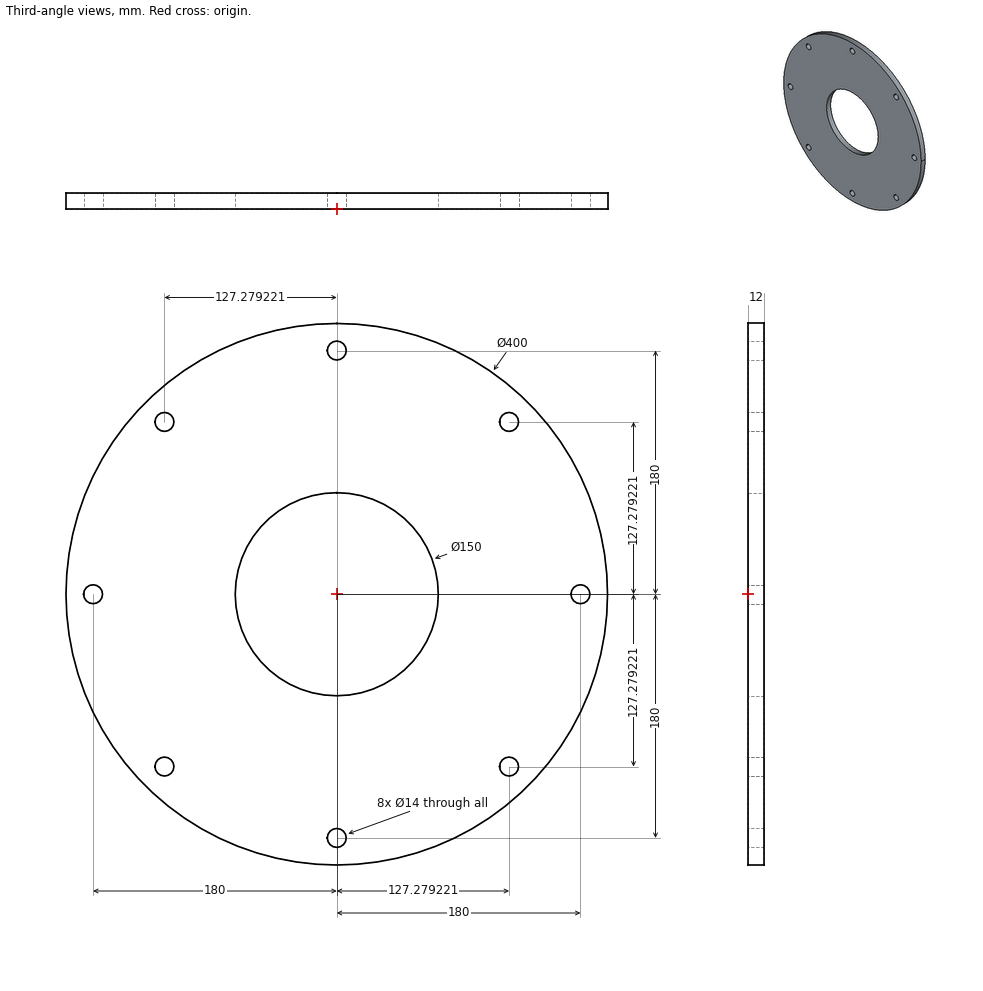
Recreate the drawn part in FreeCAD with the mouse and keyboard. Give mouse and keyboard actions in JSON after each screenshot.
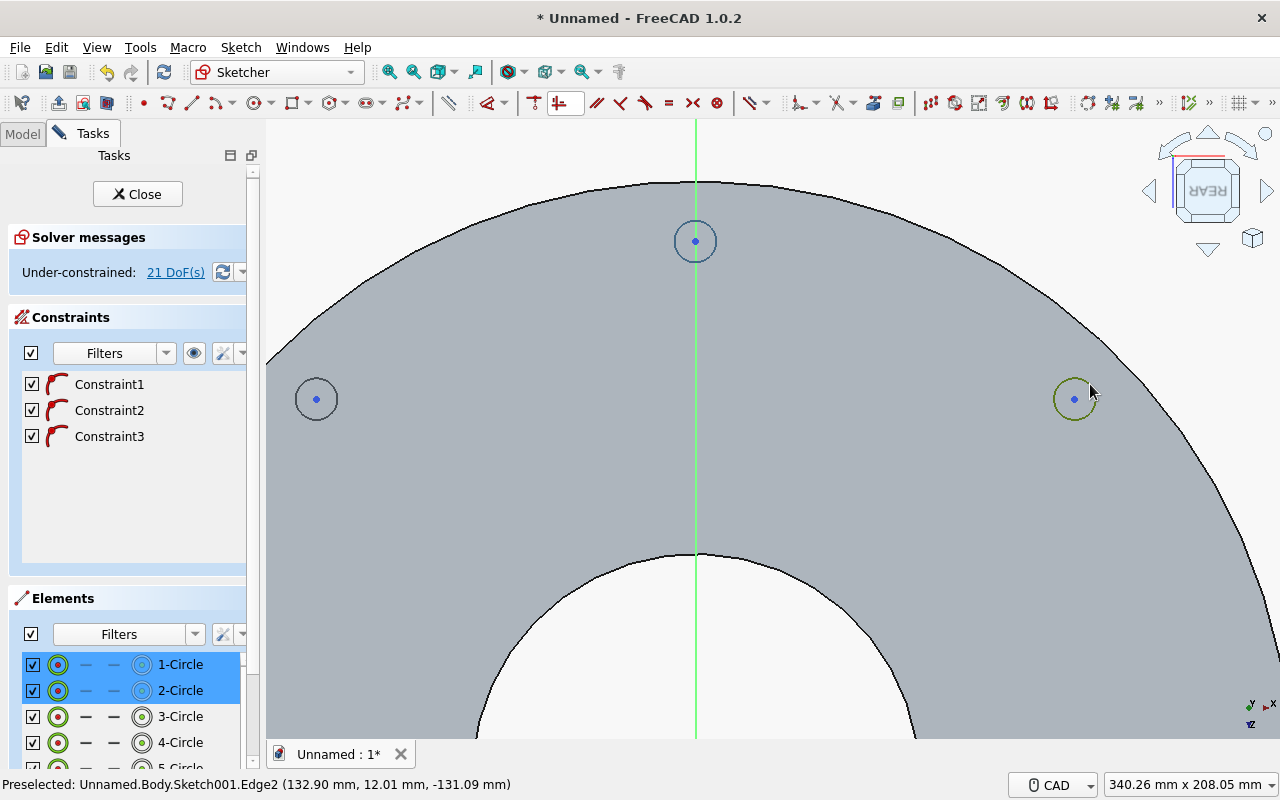
{"action": "scroll", "coordinate": [710, 226], "scroll_direction": "down", "scroll_amount": 5}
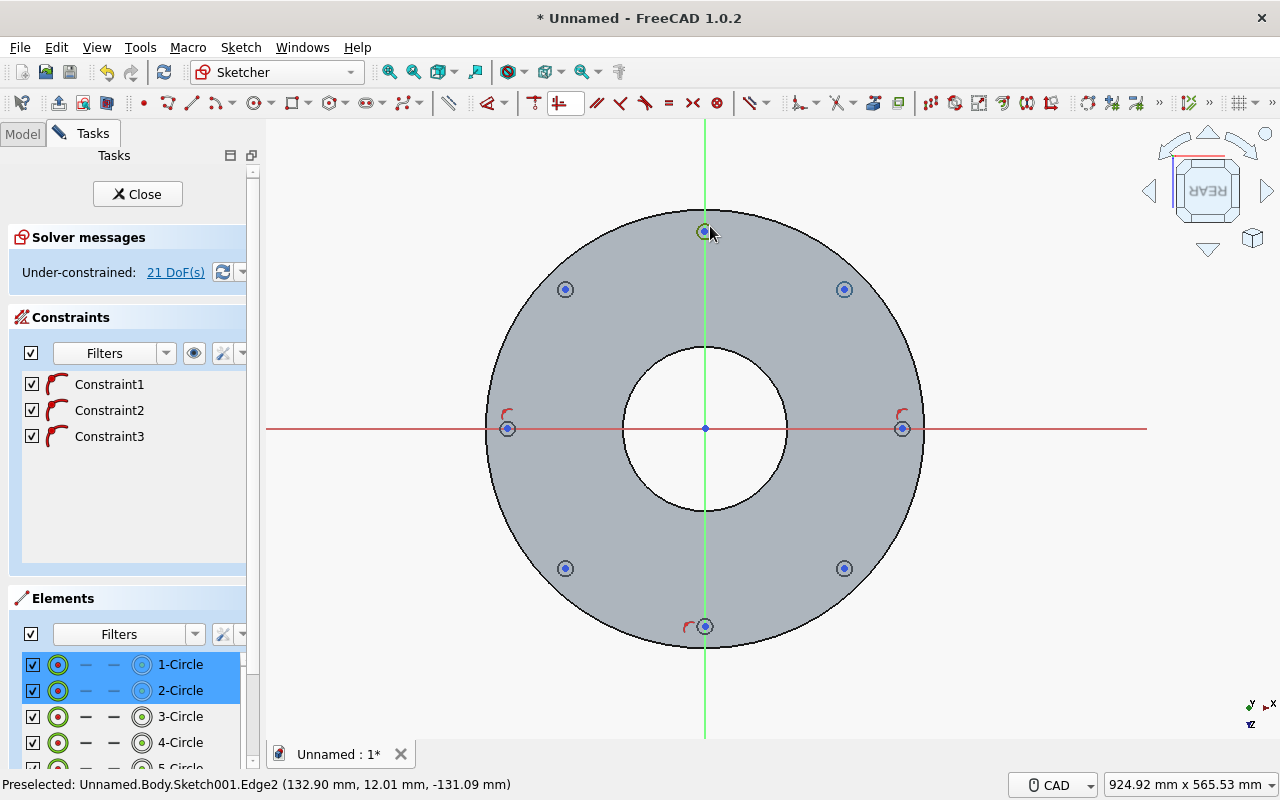
{"action": "scroll", "coordinate": [908, 424], "scroll_direction": "up", "scroll_amount": 5}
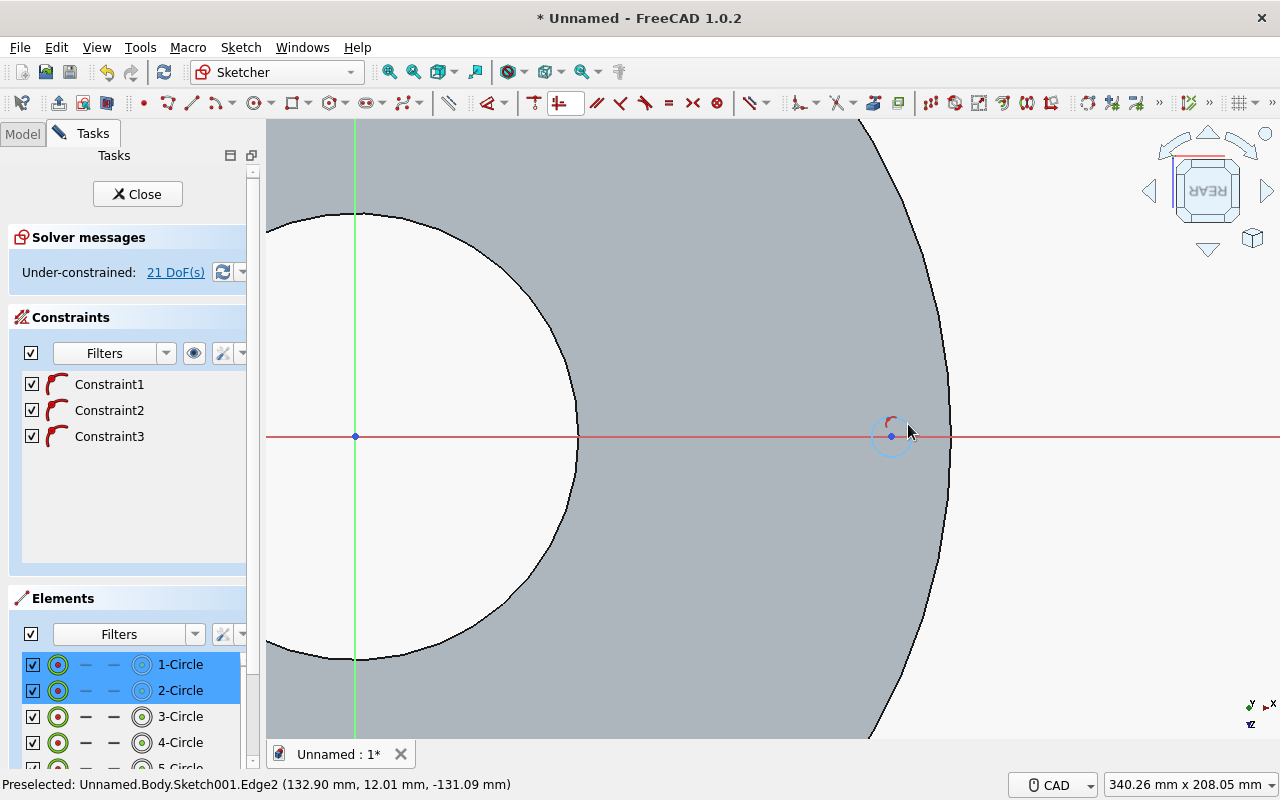
{"action": "left_click", "coordinate": [906, 422]}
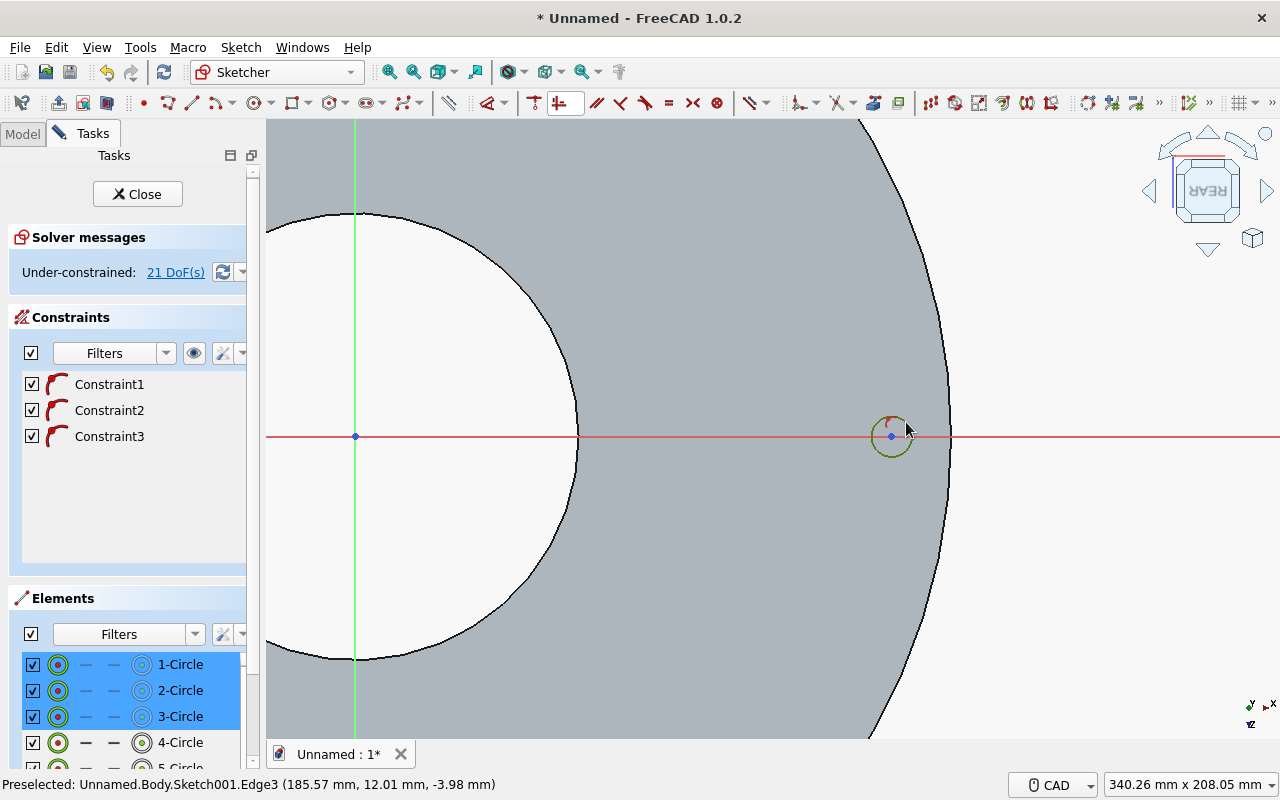
{"action": "scroll", "coordinate": [908, 424], "scroll_direction": "down", "scroll_amount": 5}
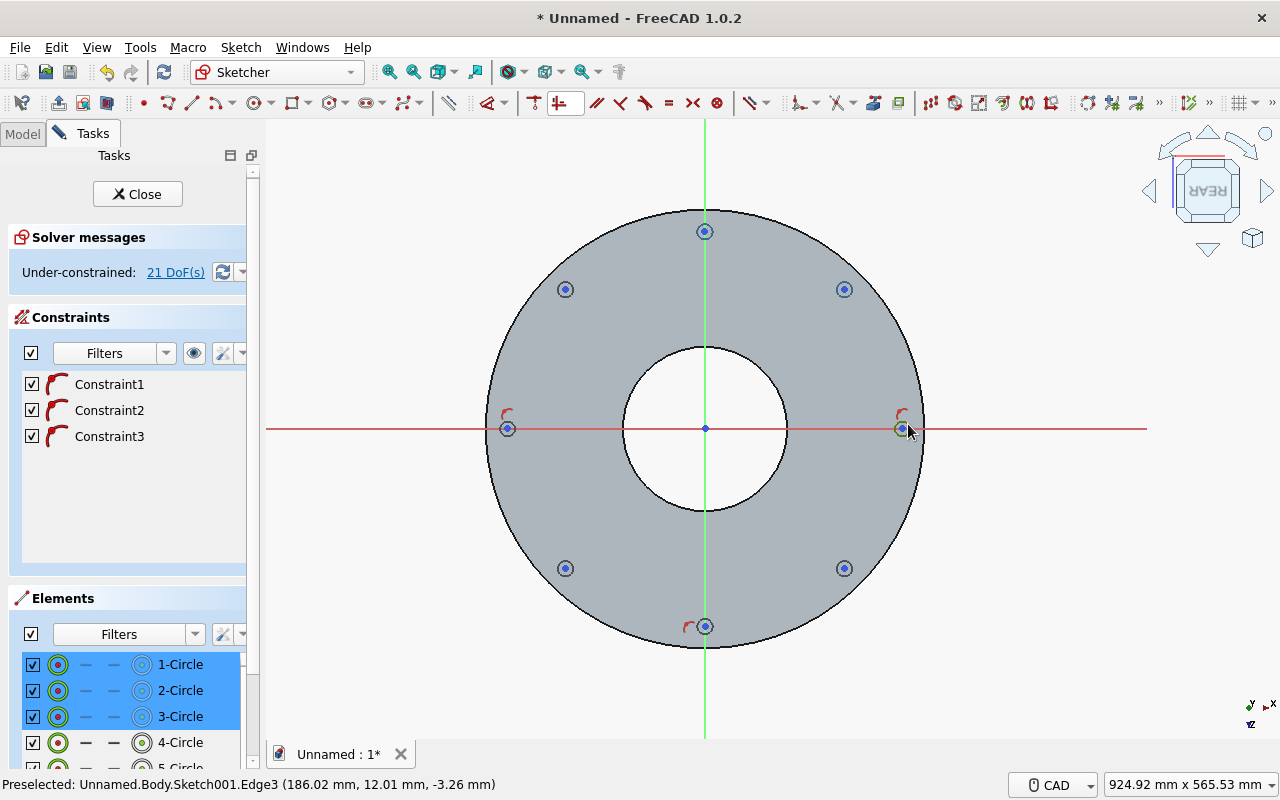
{"action": "scroll", "coordinate": [850, 563], "scroll_direction": "up", "scroll_amount": 3}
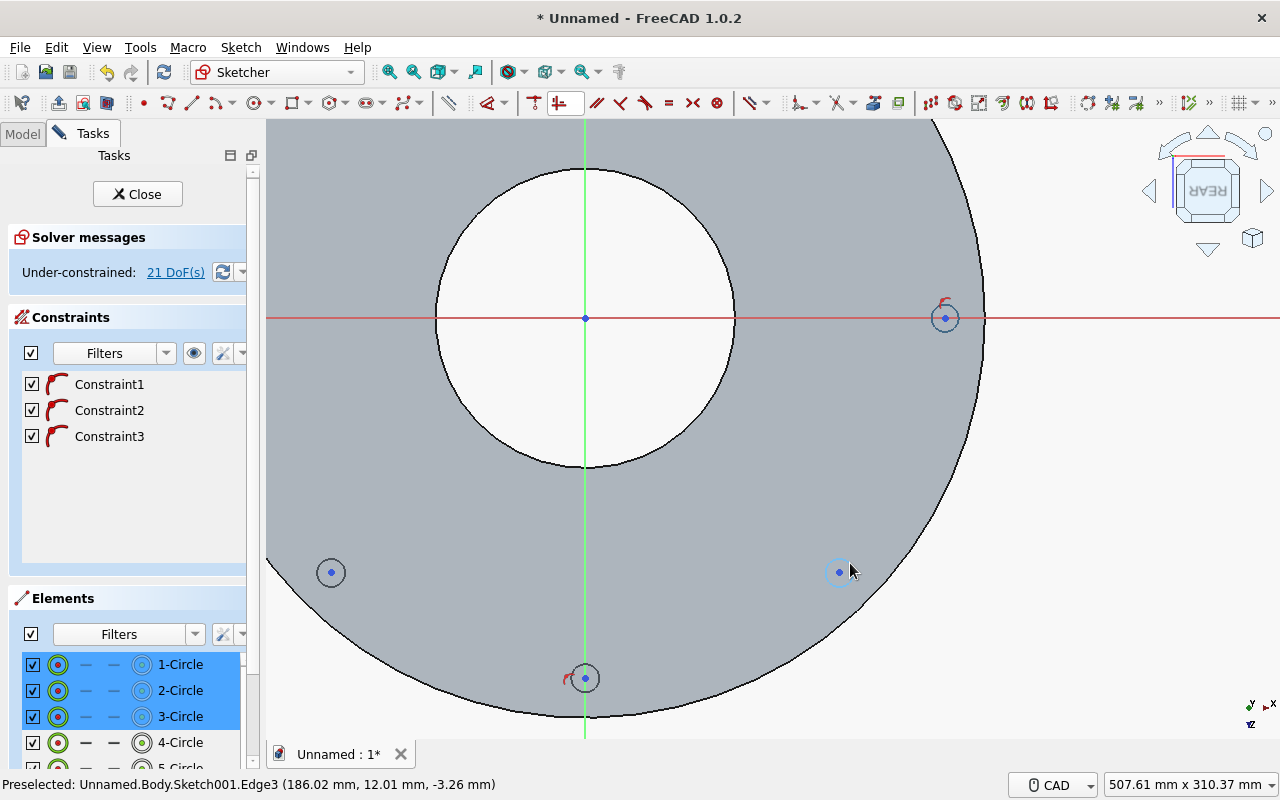
{"action": "left_click", "coordinate": [849, 563]}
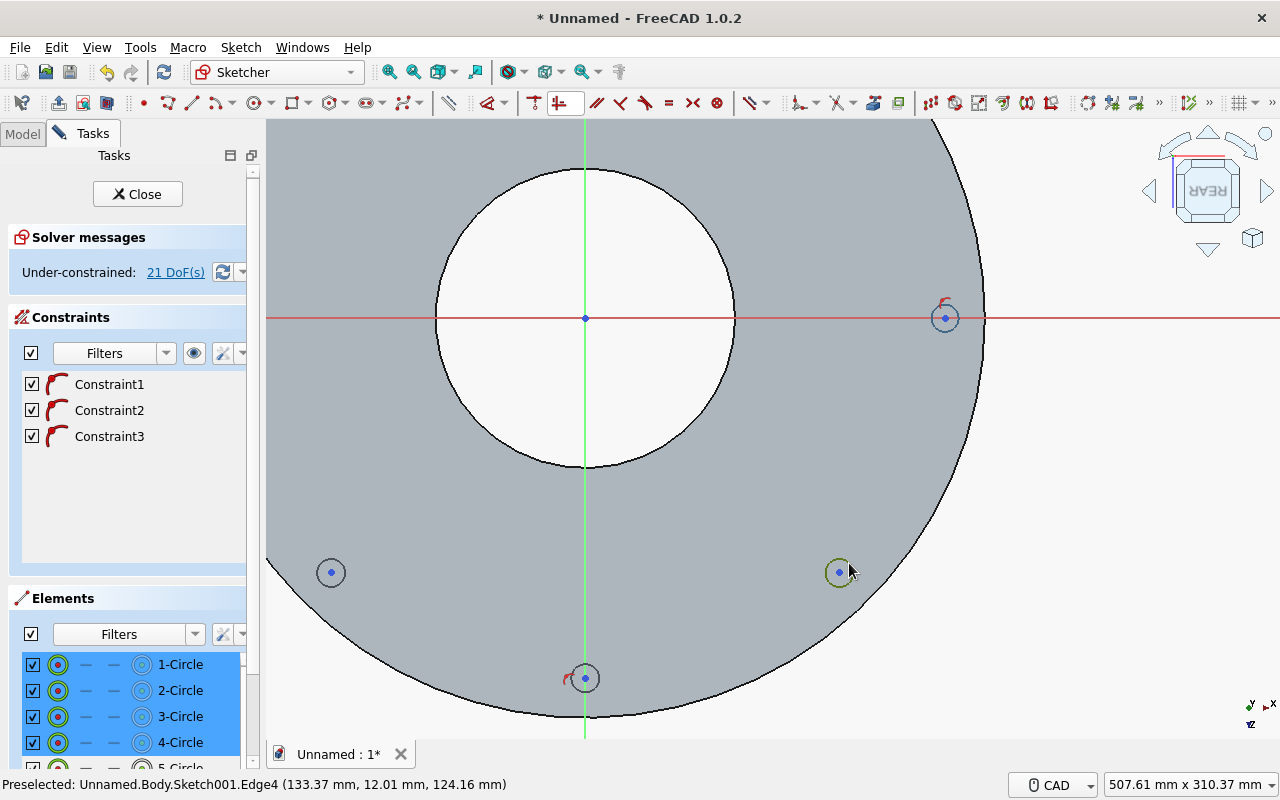
{"action": "scroll", "coordinate": [595, 668], "scroll_direction": "up", "scroll_amount": 2}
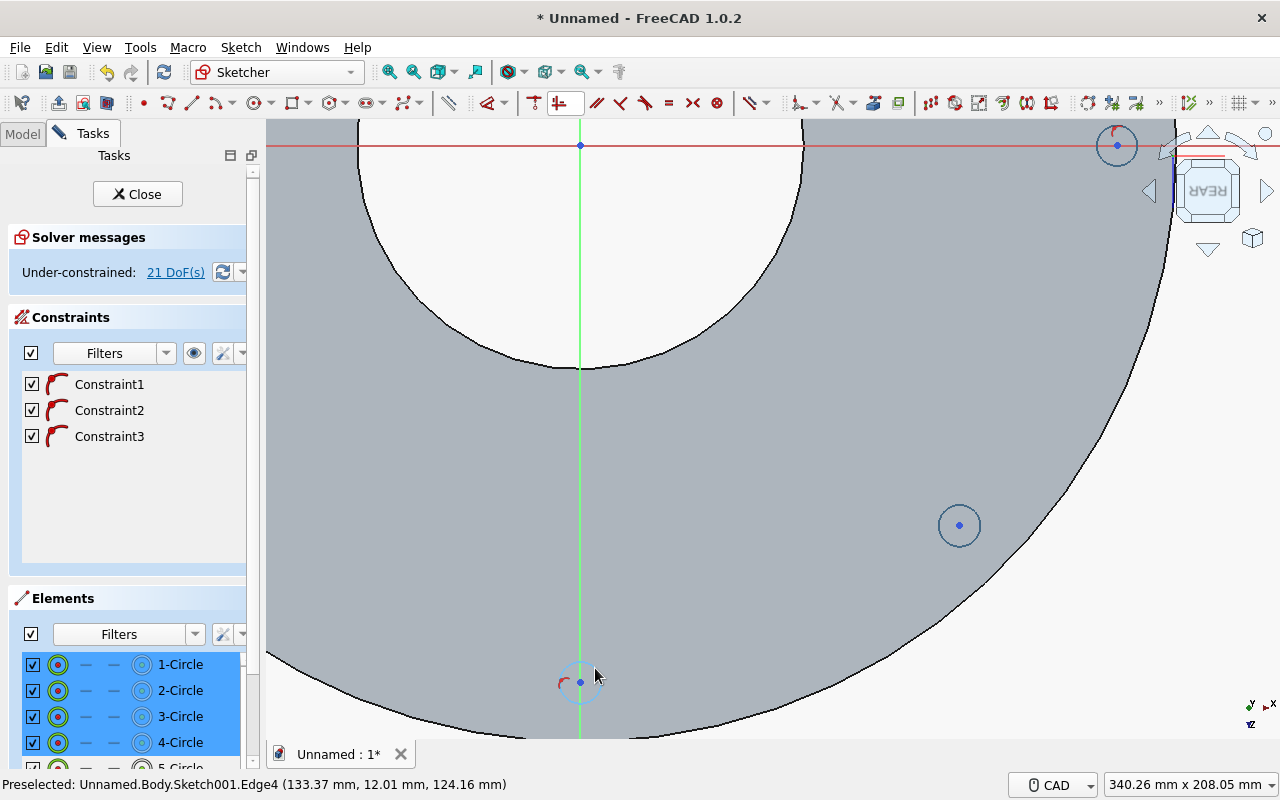
{"action": "left_click", "coordinate": [595, 668]}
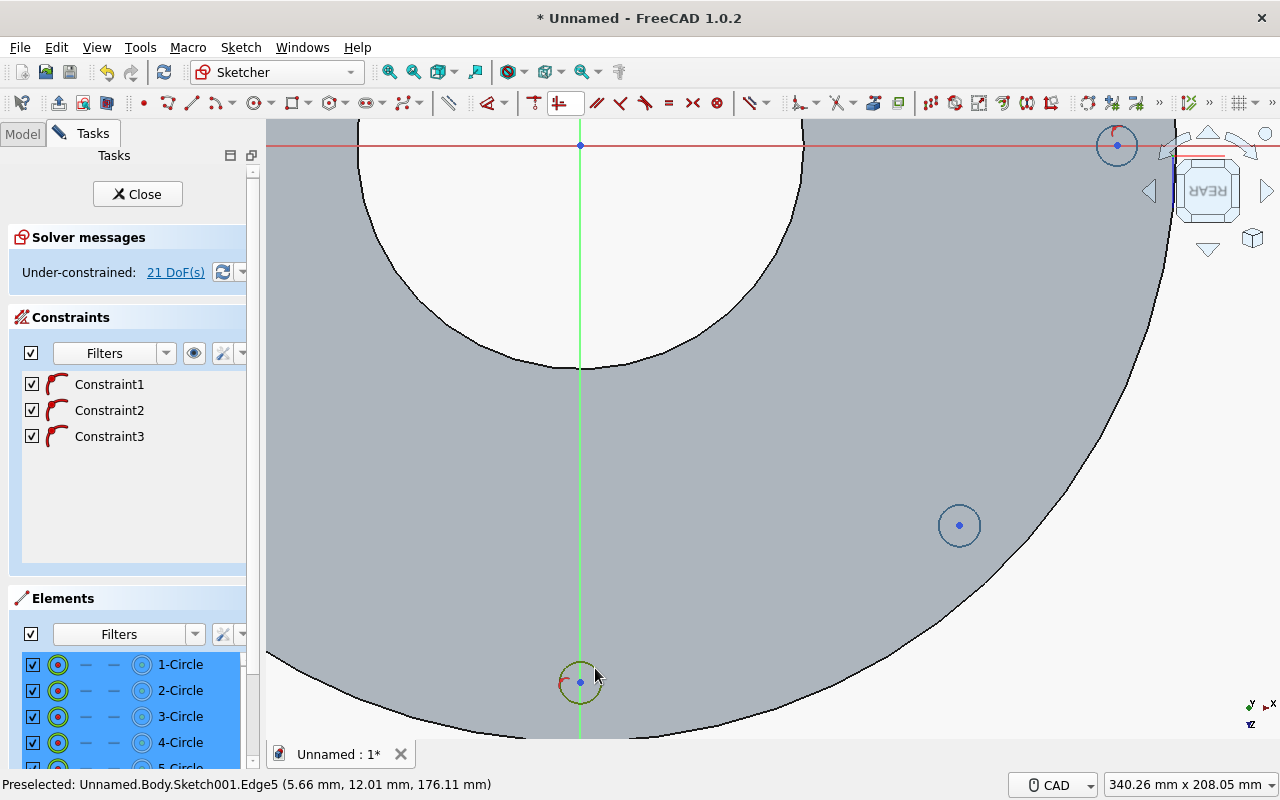
{"action": "scroll", "coordinate": [777, 594], "scroll_direction": "down", "scroll_amount": 5}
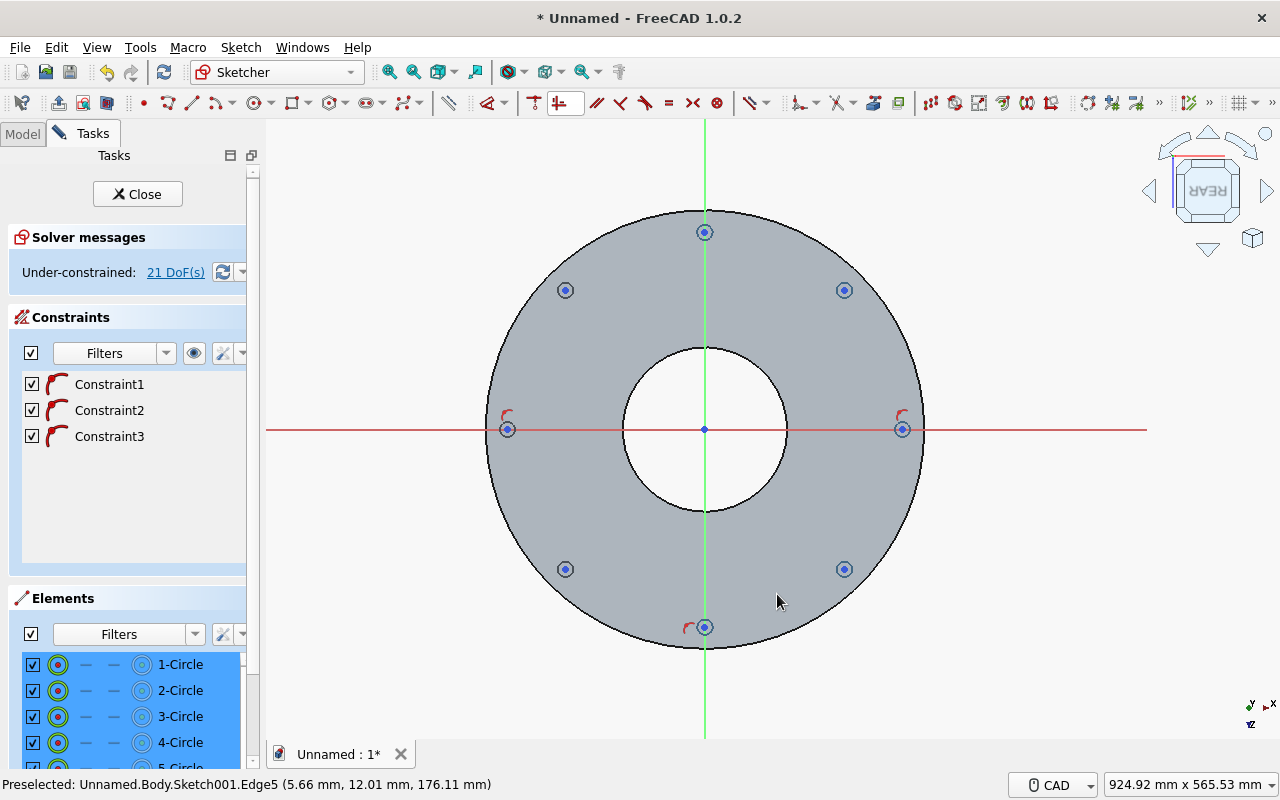
{"action": "scroll", "coordinate": [571, 564], "scroll_direction": "up", "scroll_amount": 3}